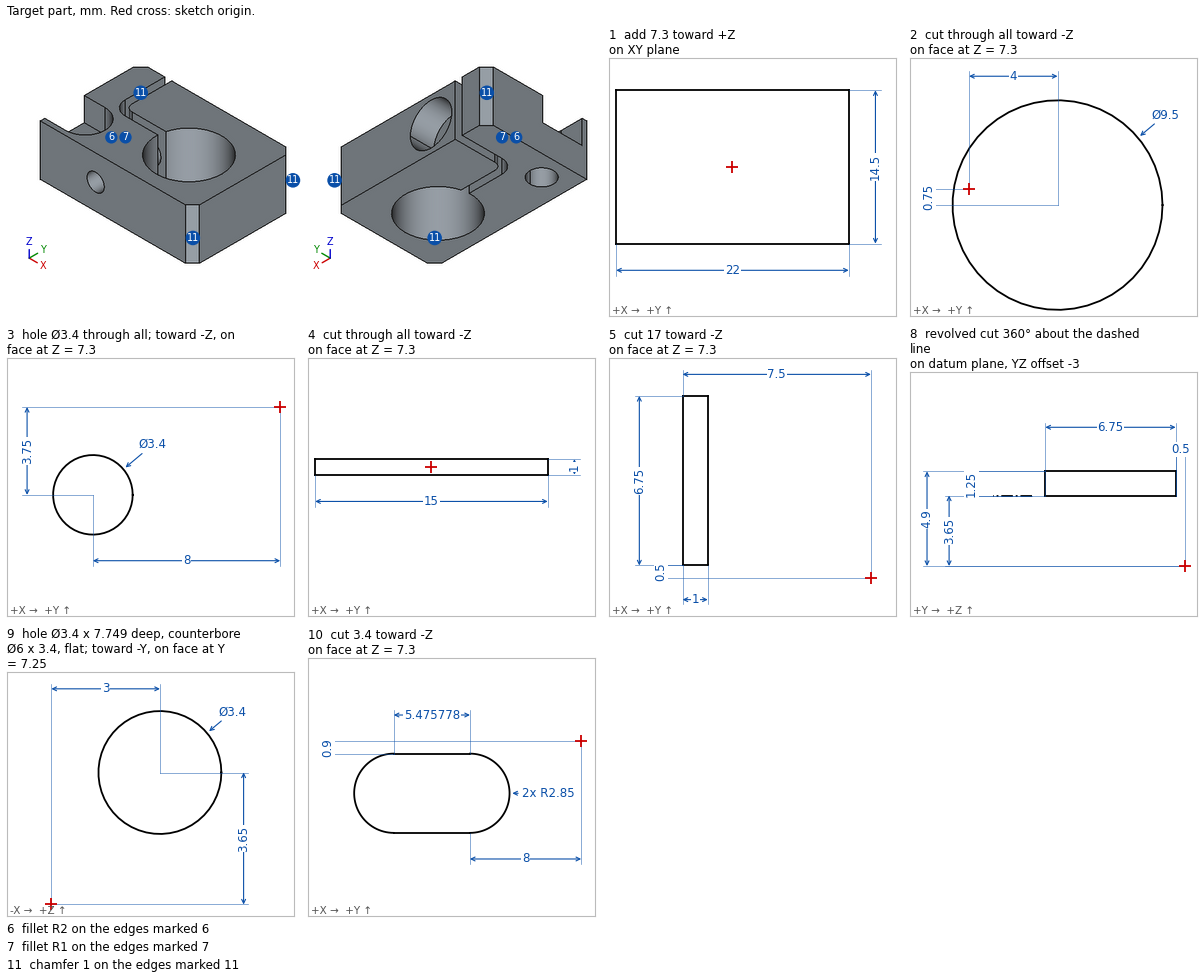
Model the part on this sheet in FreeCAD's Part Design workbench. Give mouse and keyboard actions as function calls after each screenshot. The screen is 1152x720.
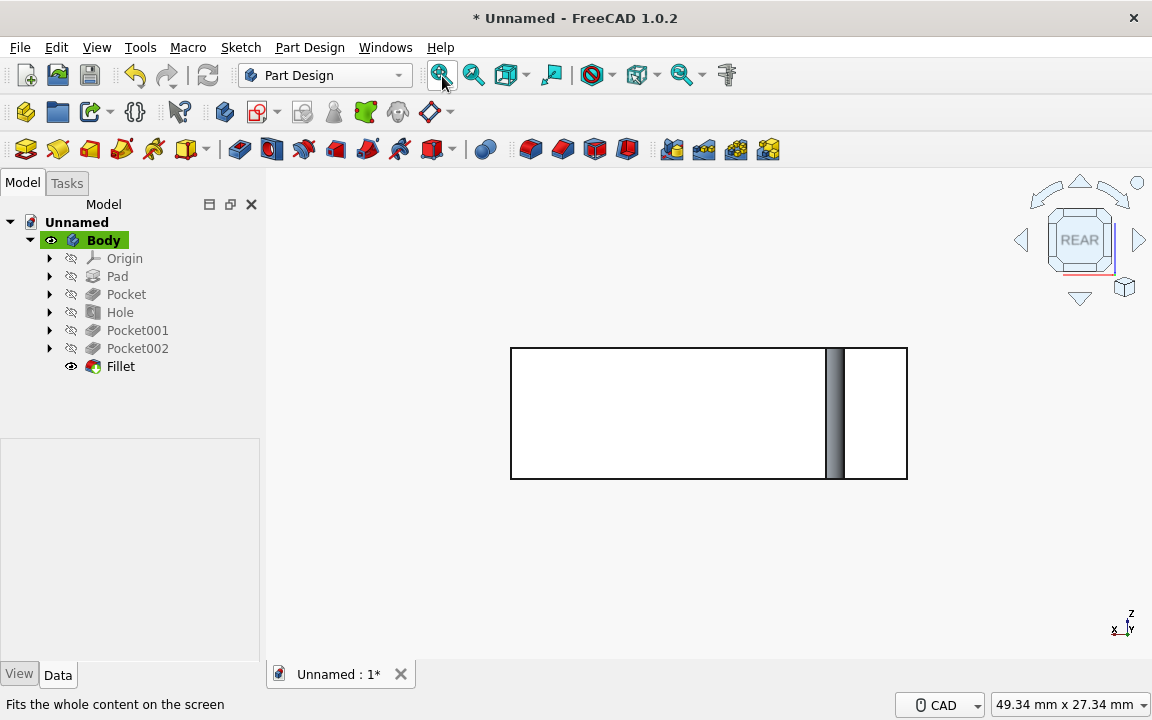
key(6)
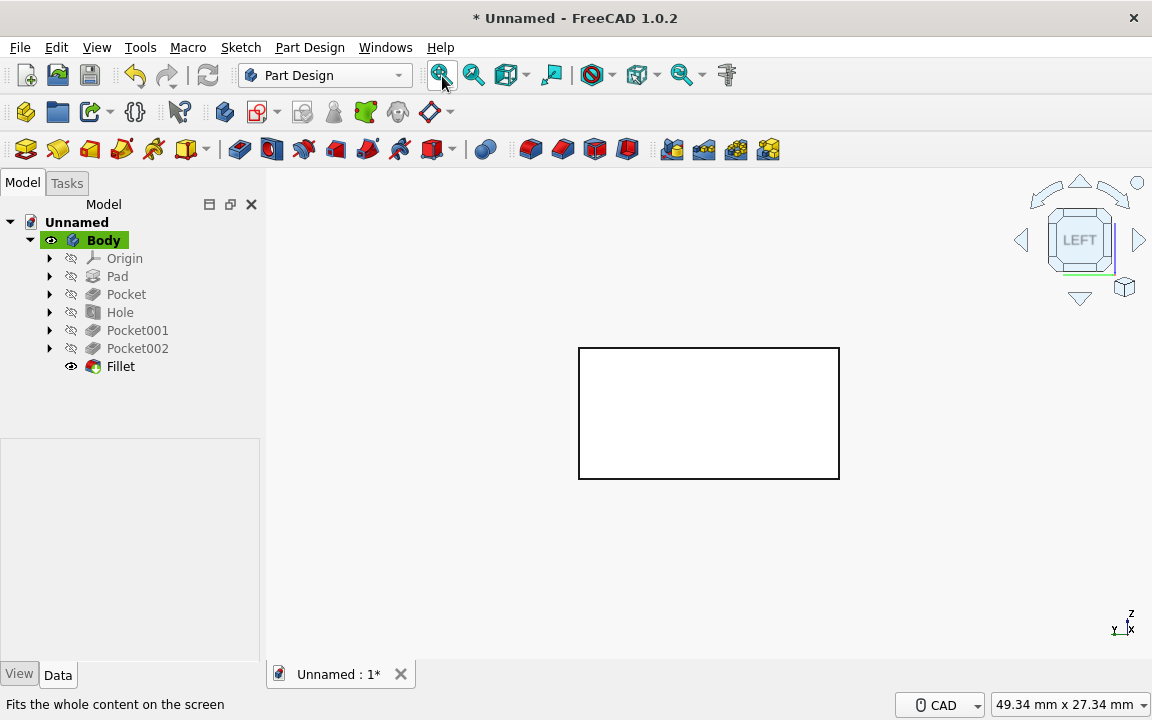
click(442, 76)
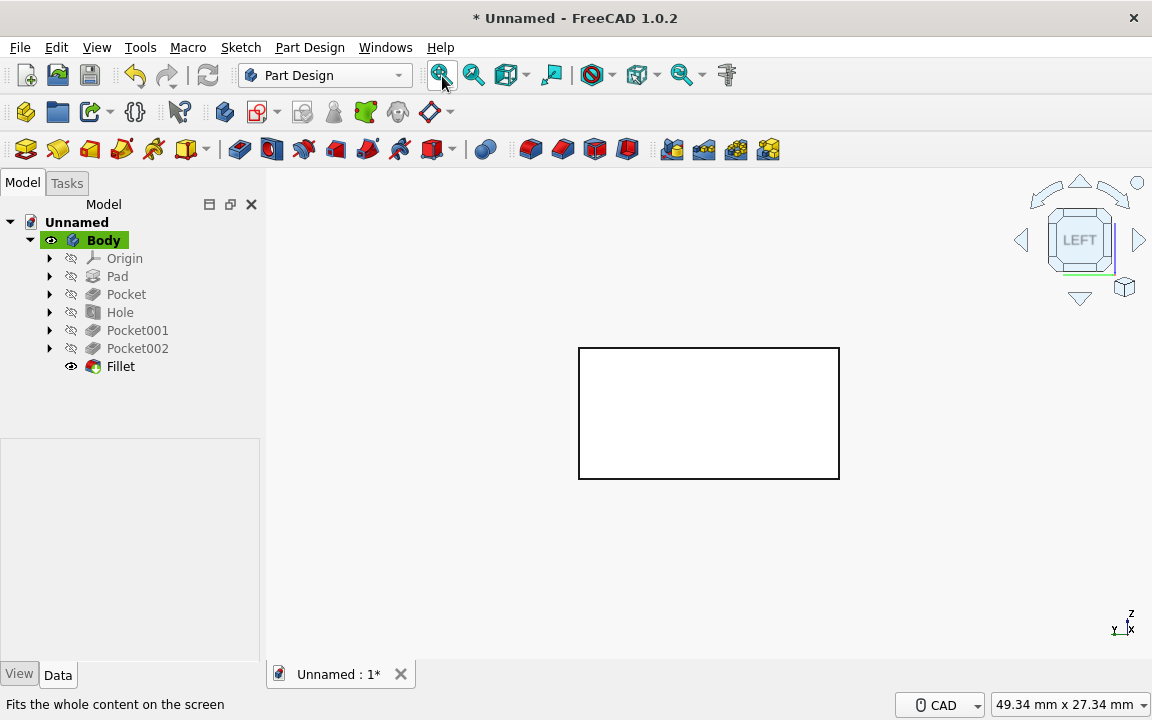
key(v)
key(3)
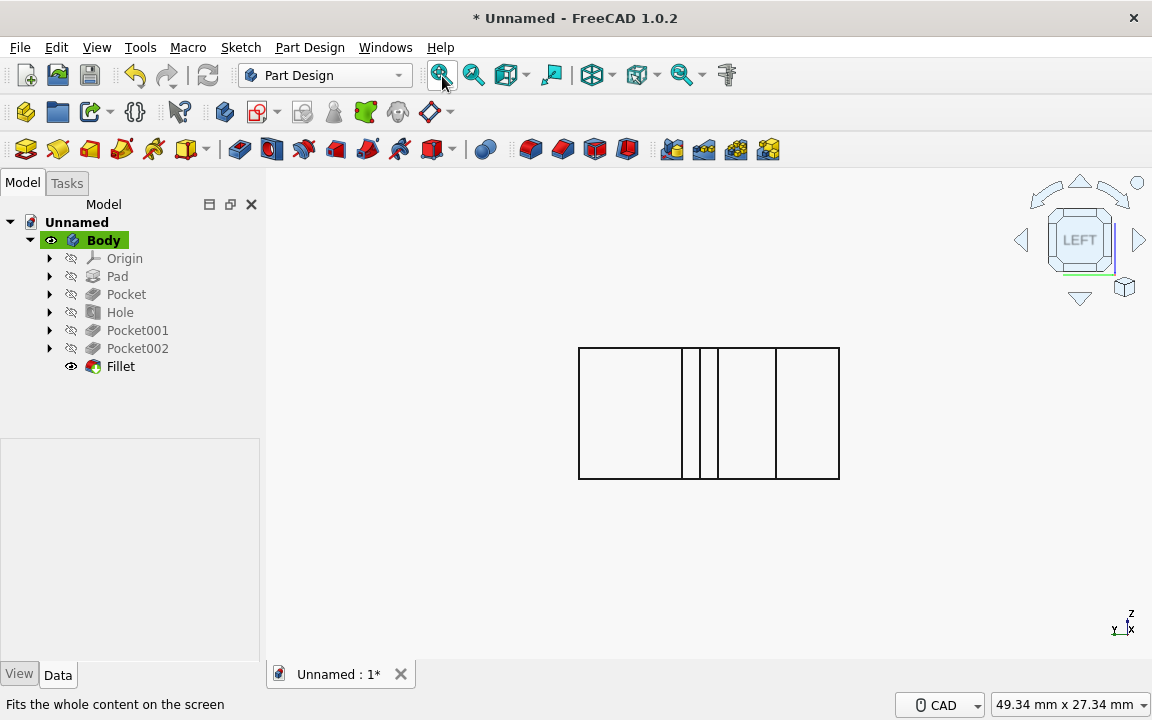
key(0)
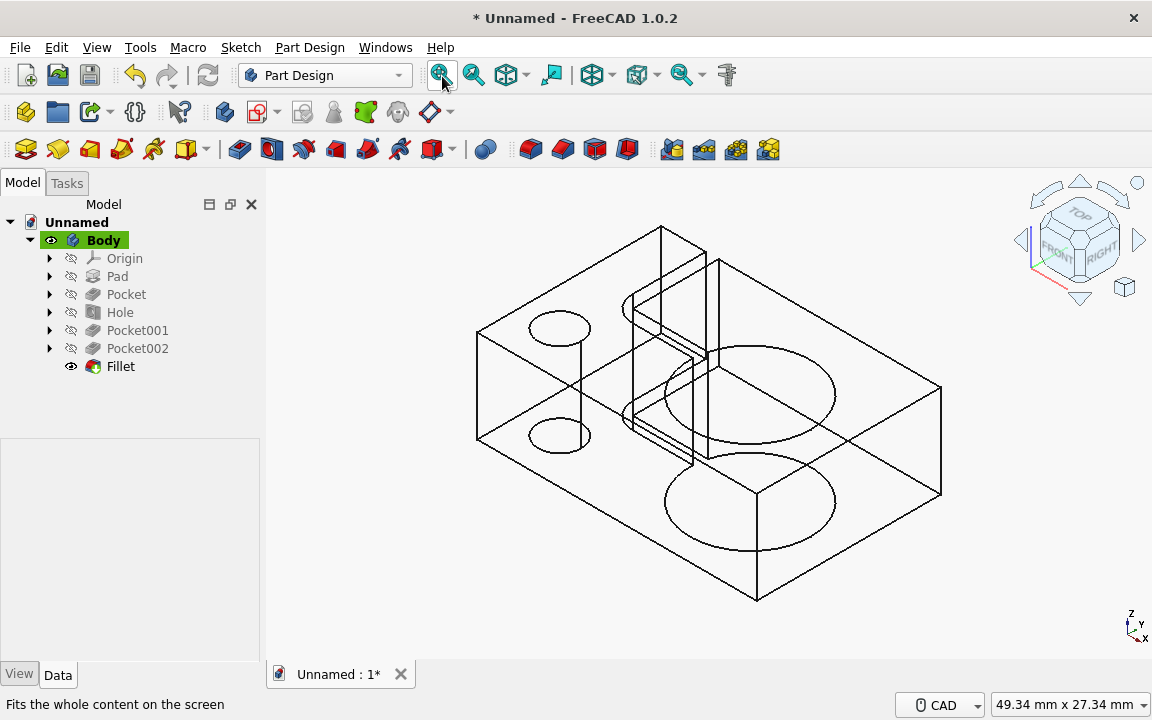
key(2)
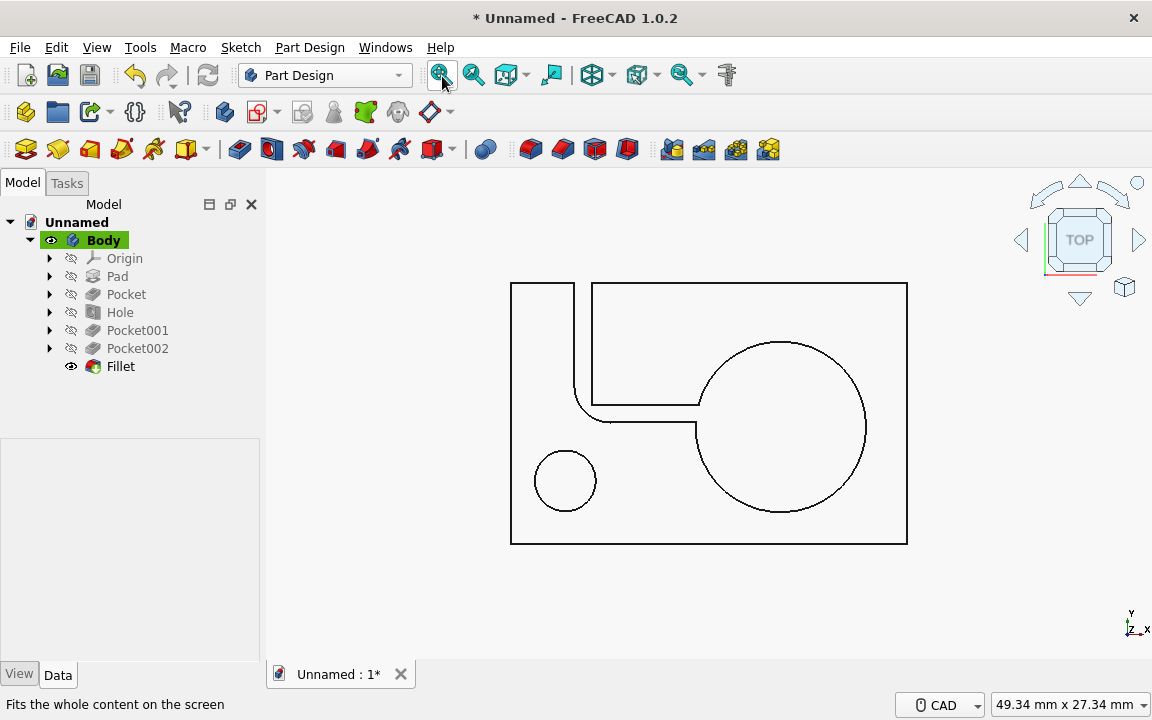
key(1)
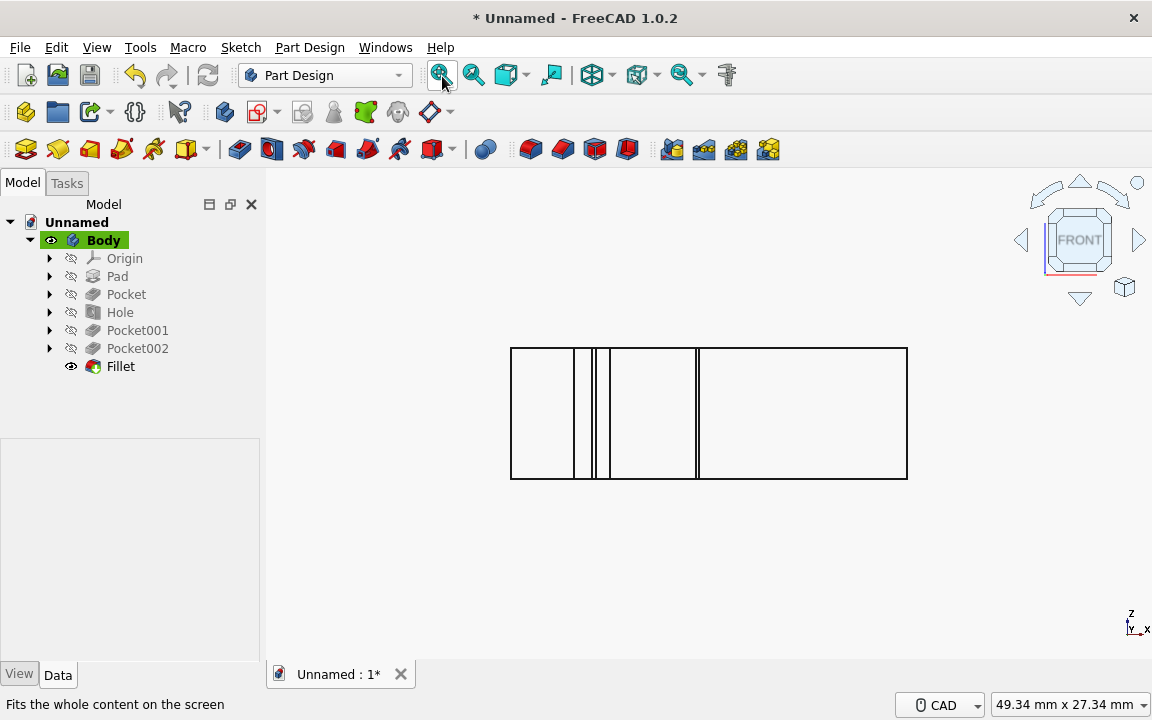
click(442, 76)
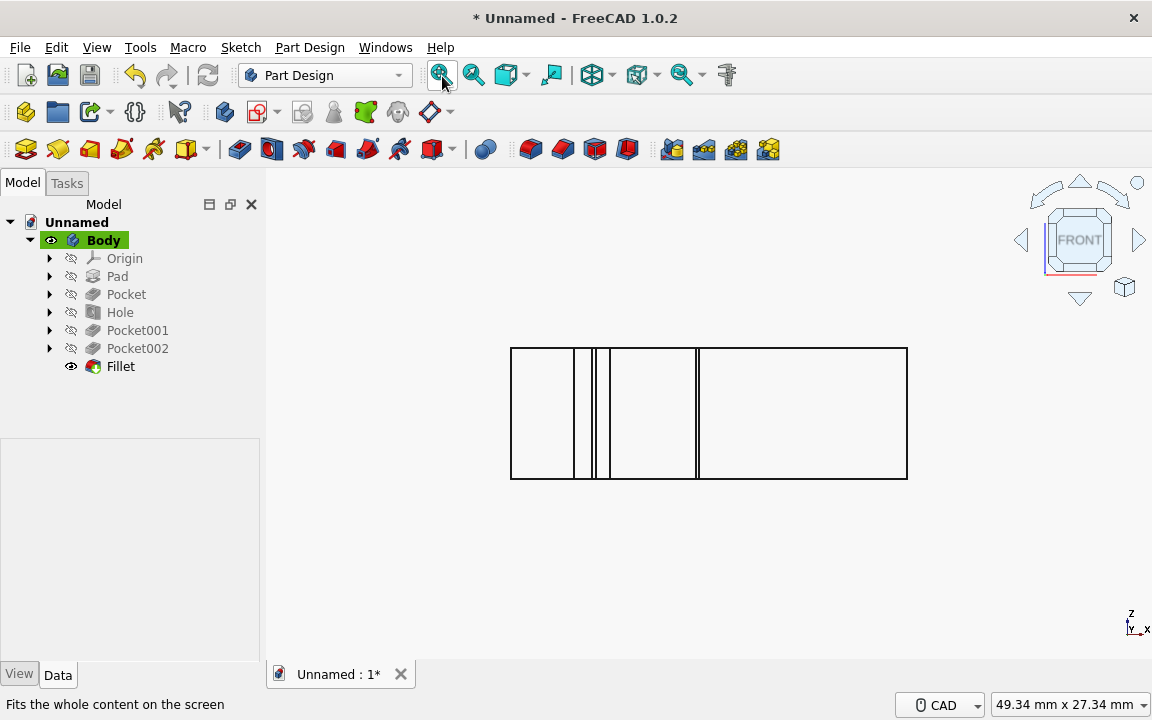
key(3)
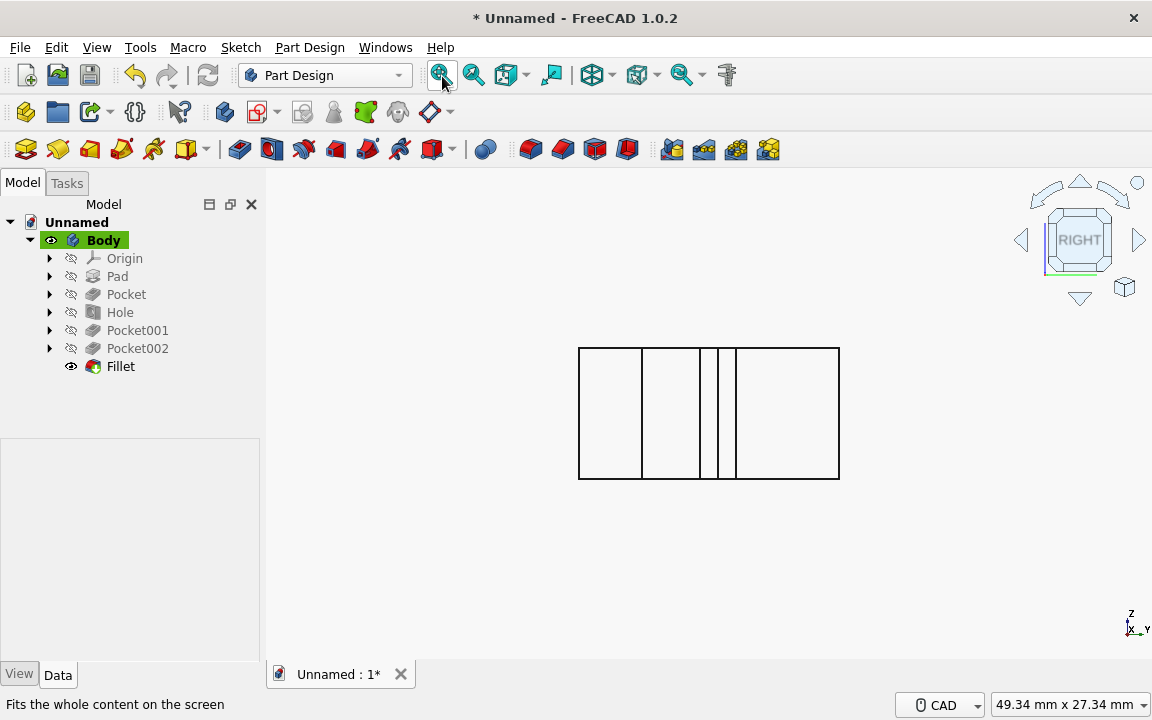
click(442, 76)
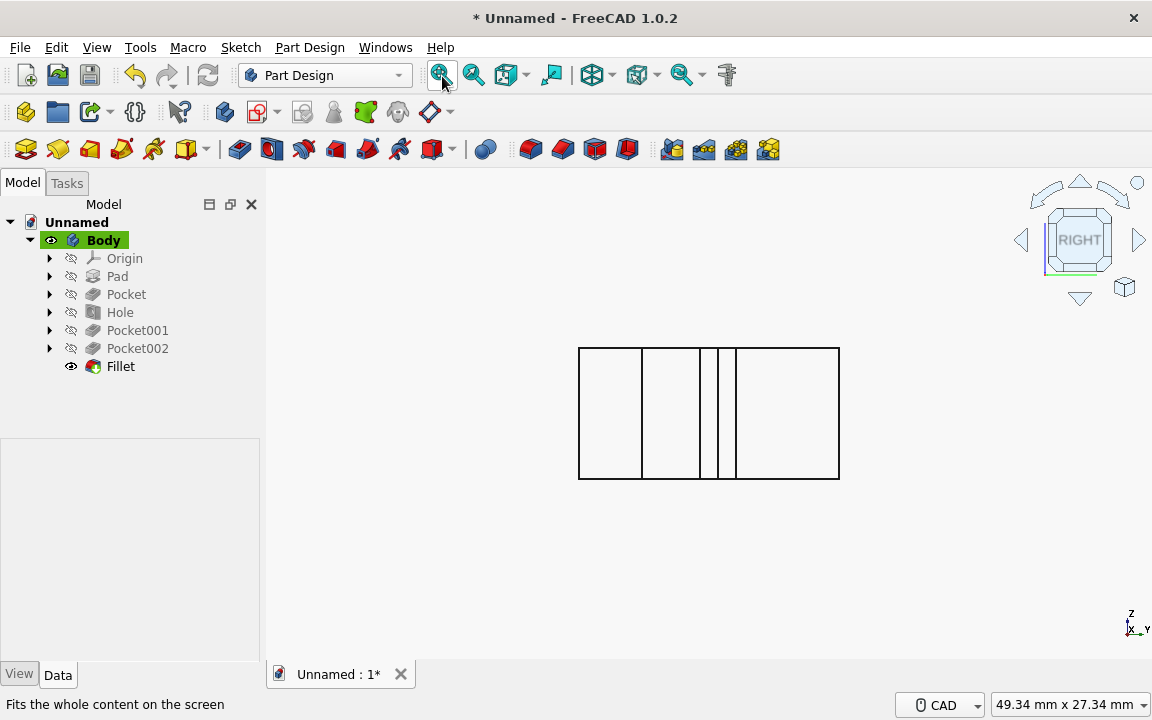
key(5)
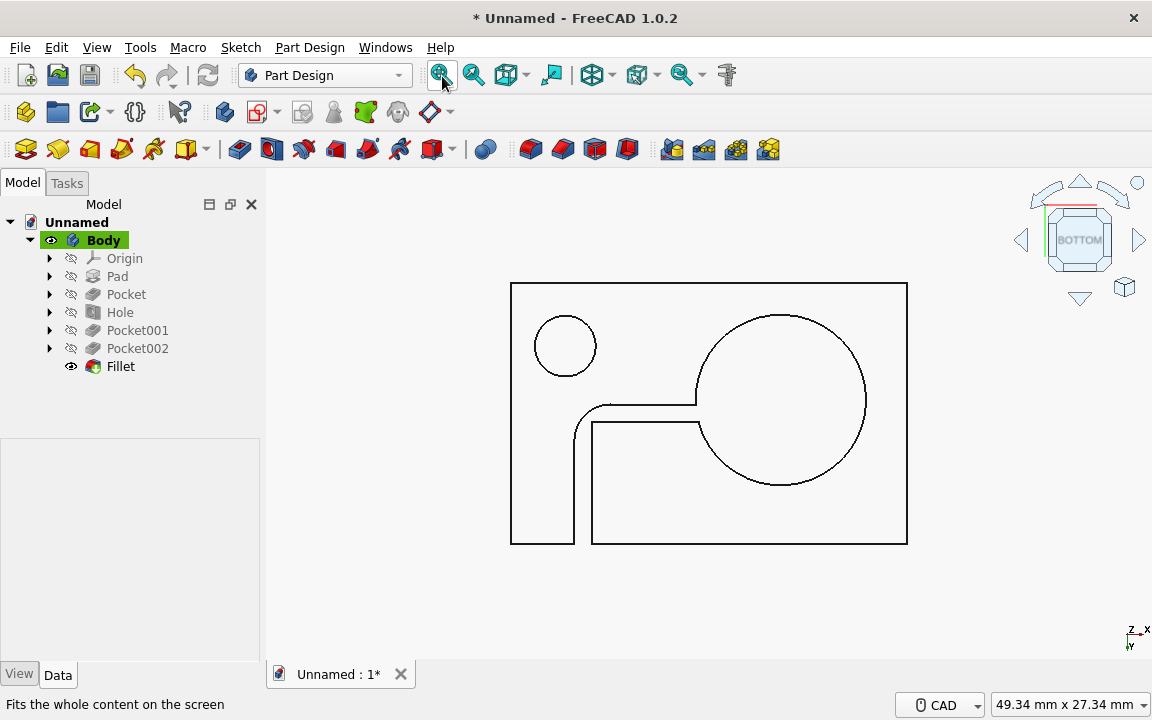
key(4)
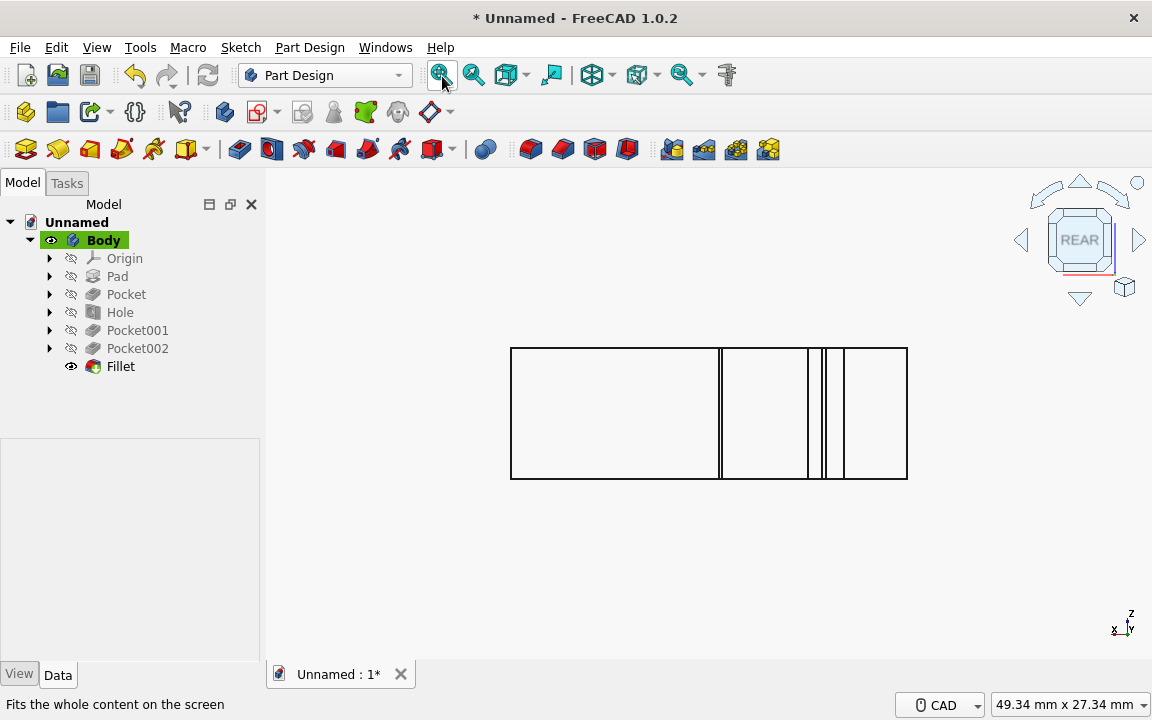
key(v)
key(f)